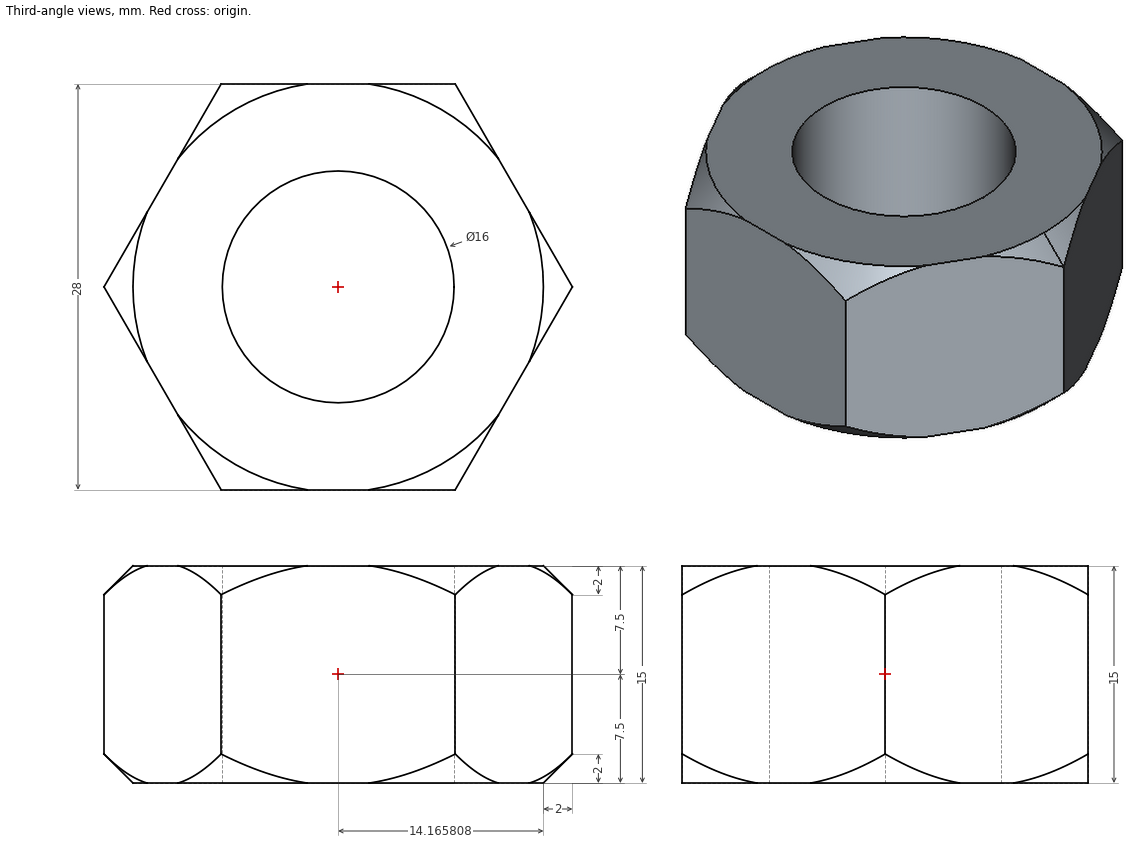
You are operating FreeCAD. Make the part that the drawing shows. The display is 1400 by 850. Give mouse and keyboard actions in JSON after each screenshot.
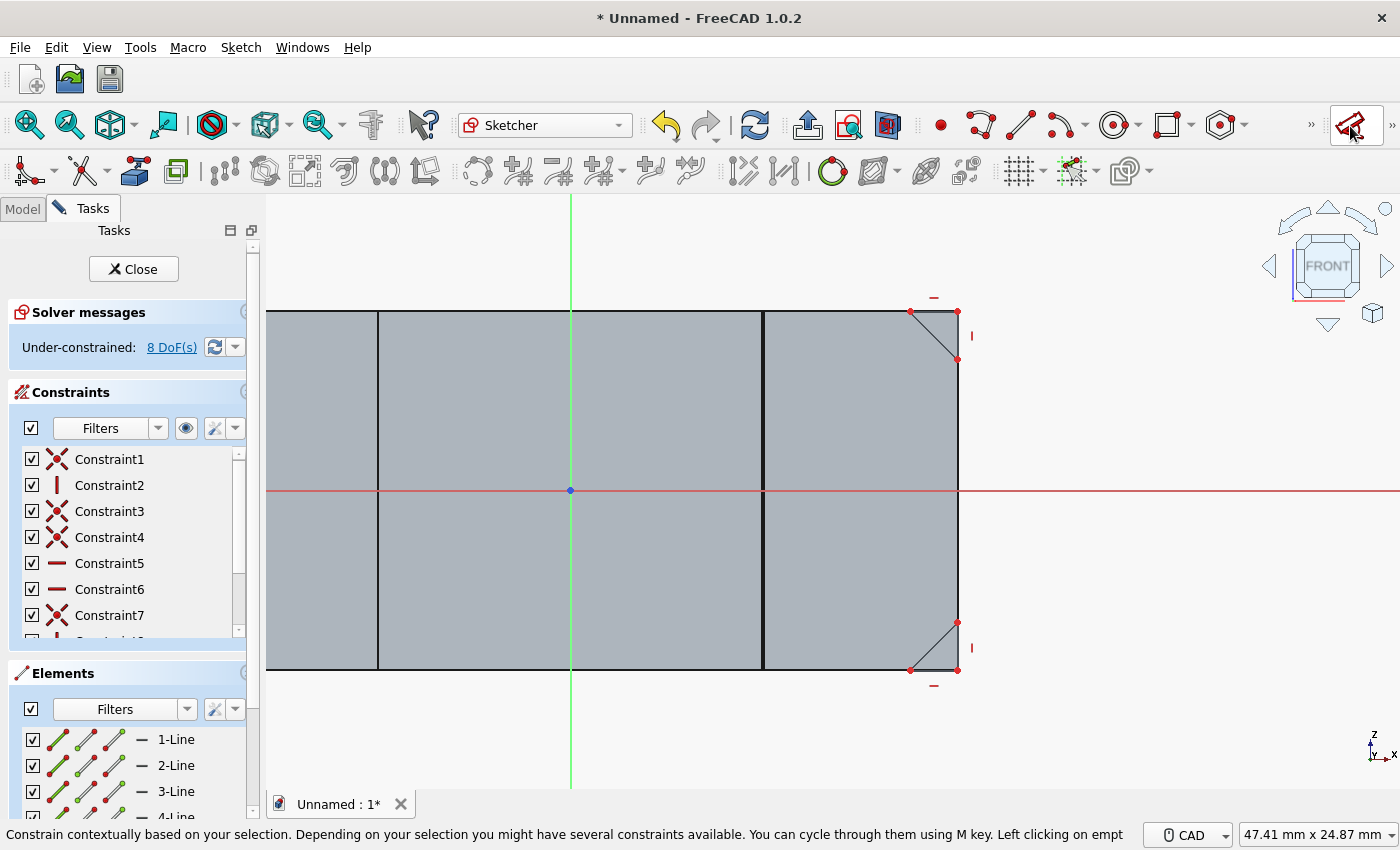
{"action": "scroll", "coordinate": [958, 637], "scroll_direction": "up", "scroll_amount": 2}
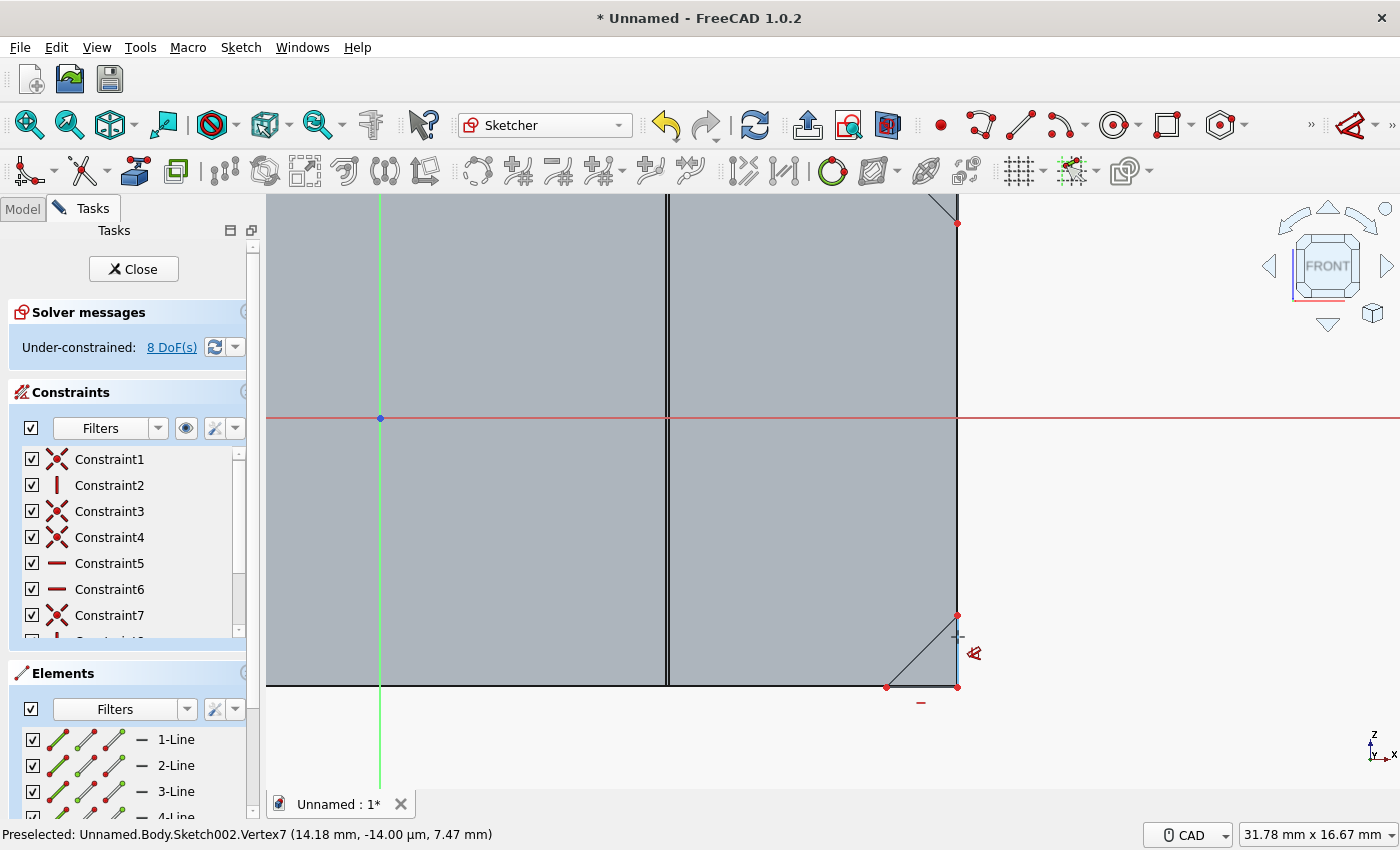
{"action": "left_click", "coordinate": [958, 637]}
{"action": "left_click", "coordinate": [992, 652]}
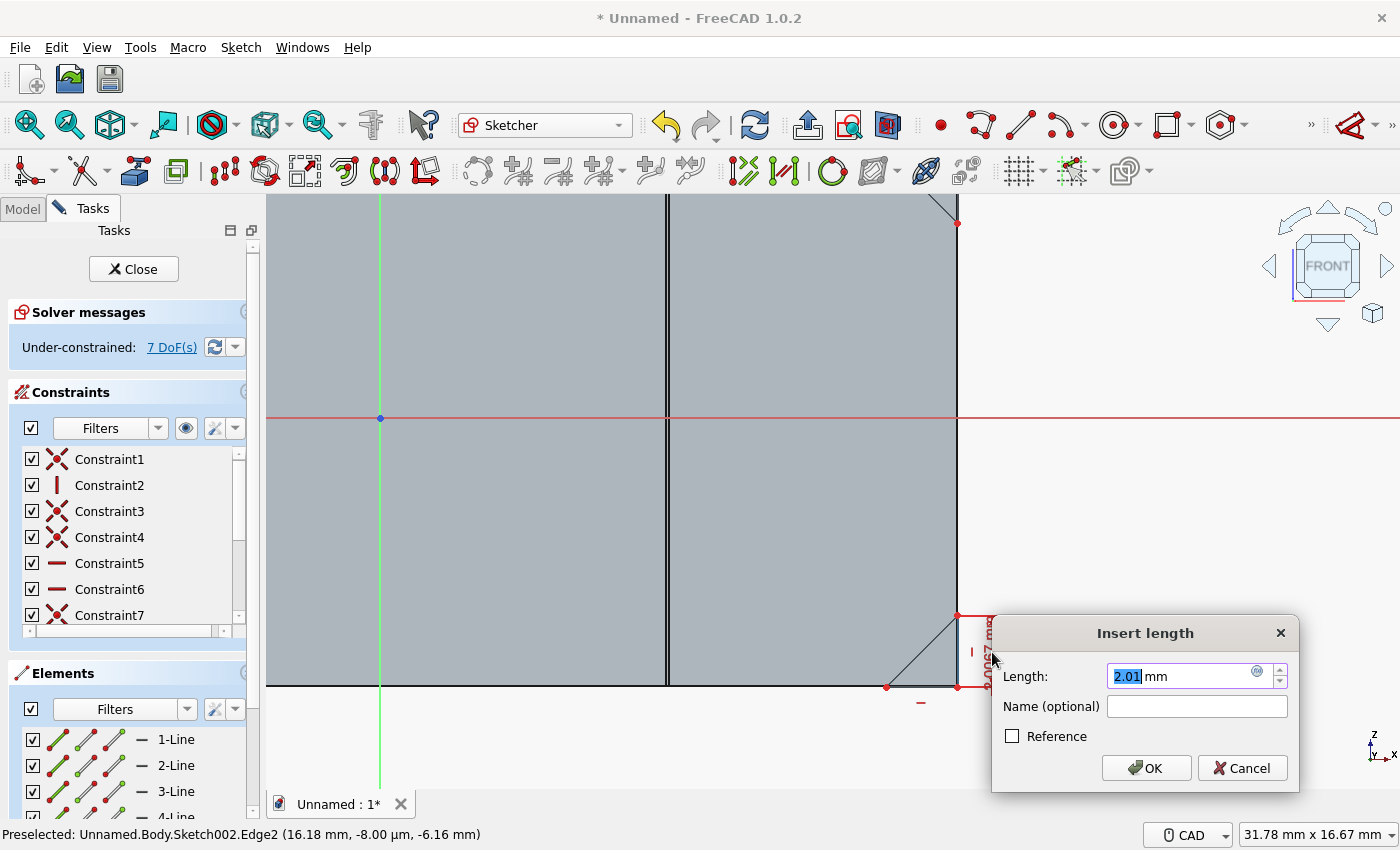
{"action": "type", "text": "2"}
{"action": "key", "text": "Return"}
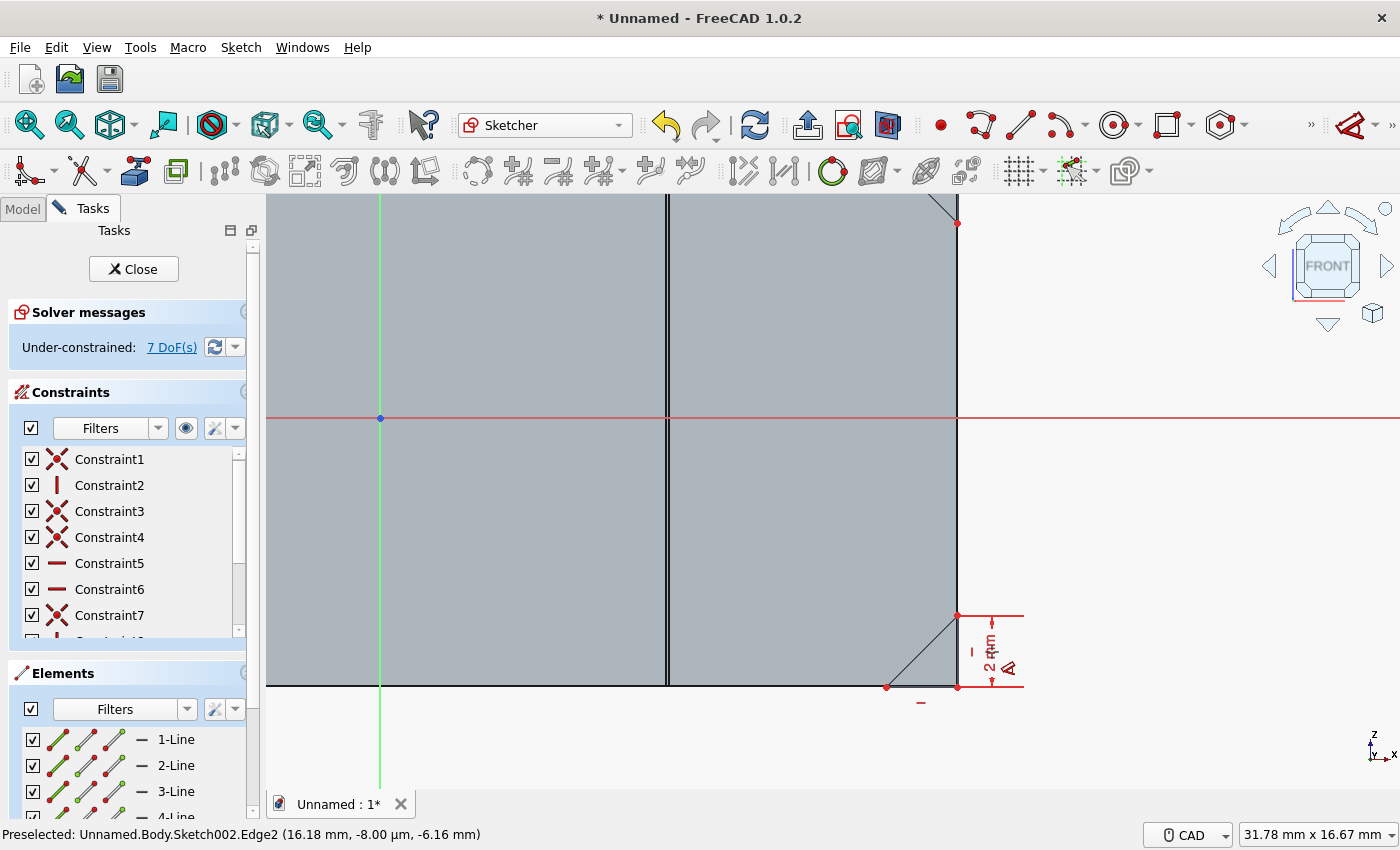
{"action": "left_click", "coordinate": [936, 687]}
{"action": "left_click", "coordinate": [922, 721]}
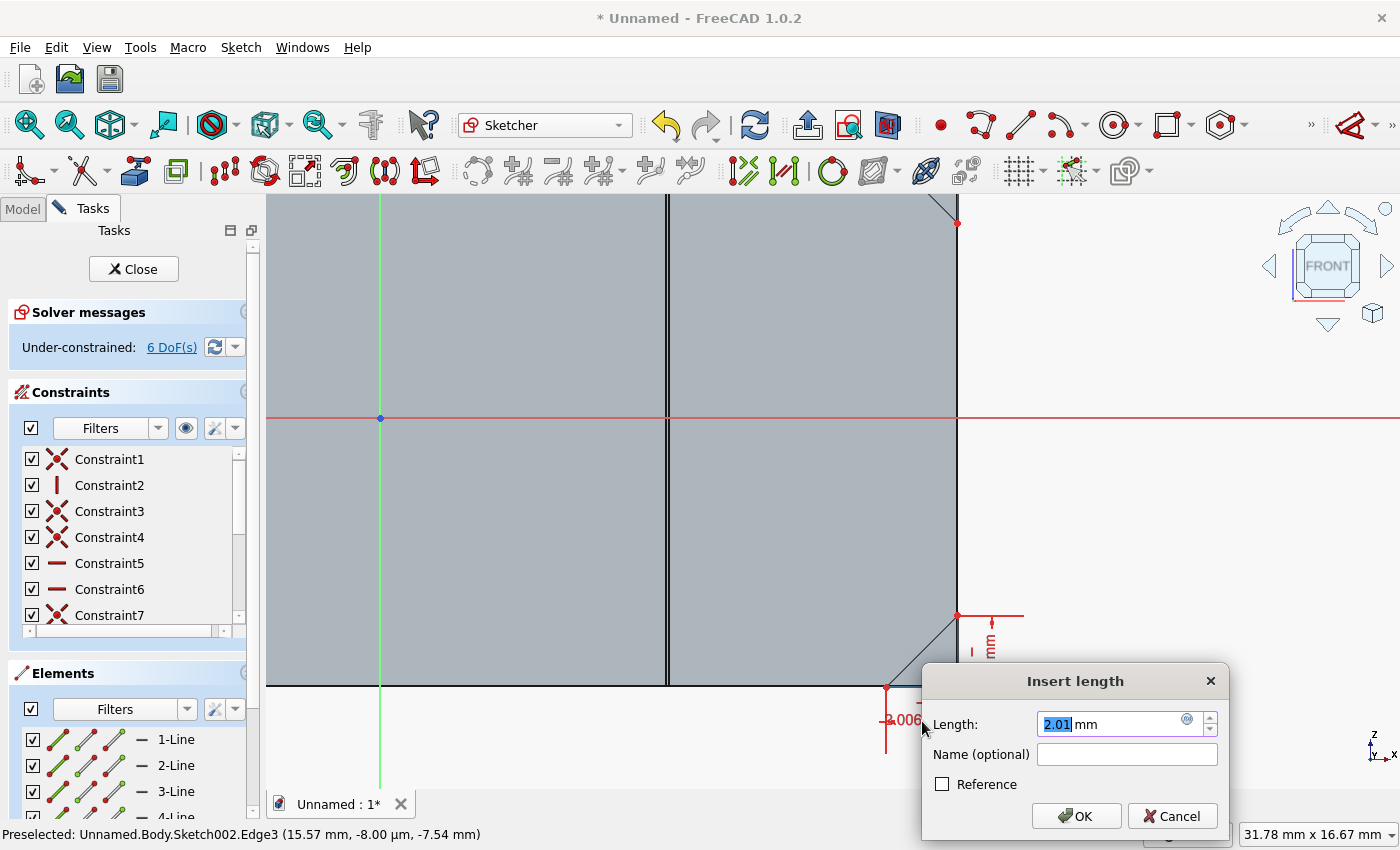
{"action": "type", "text": "2"}
{"action": "key", "text": "Return"}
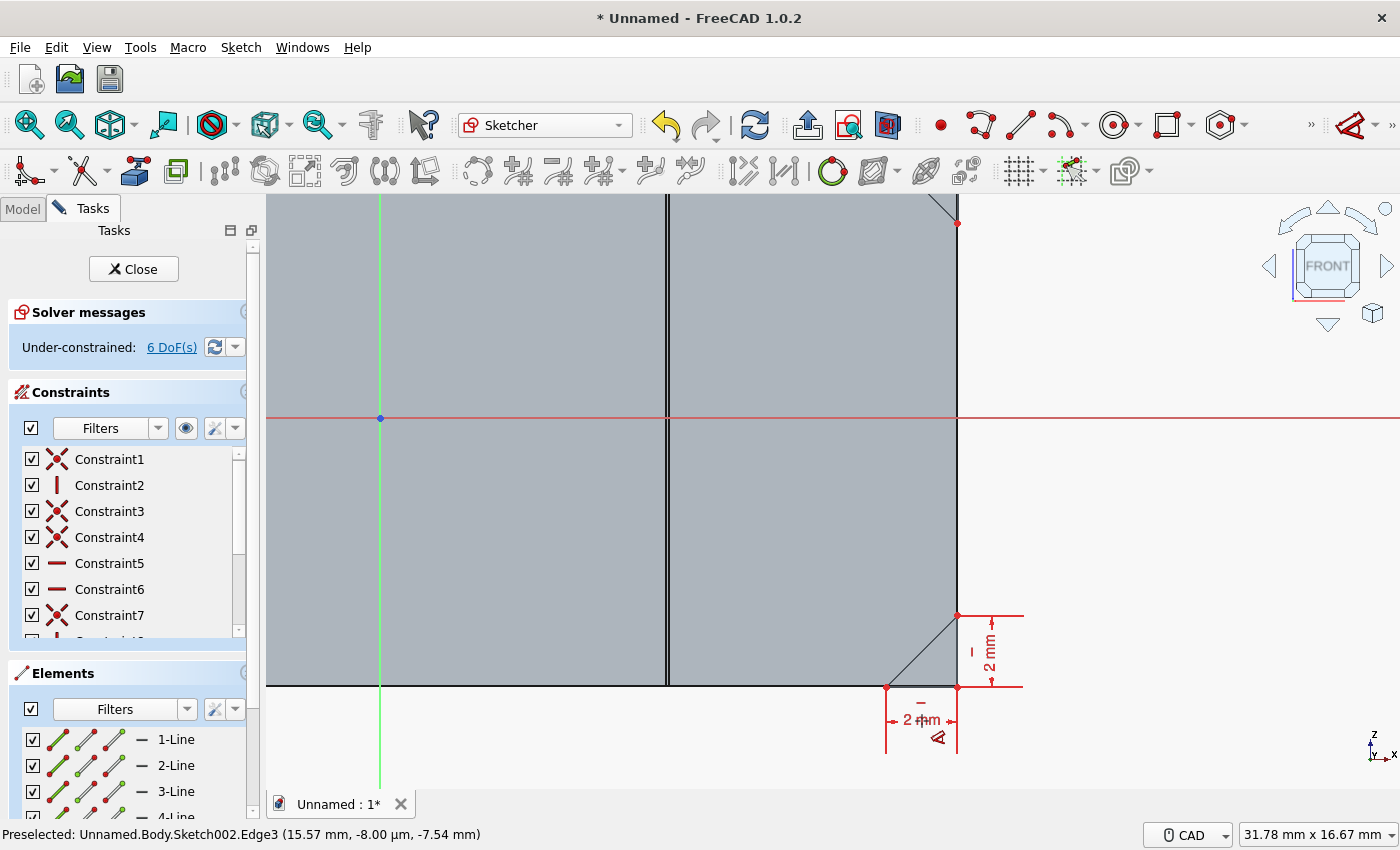
{"action": "scroll", "coordinate": [959, 640], "scroll_direction": "down", "scroll_amount": 2}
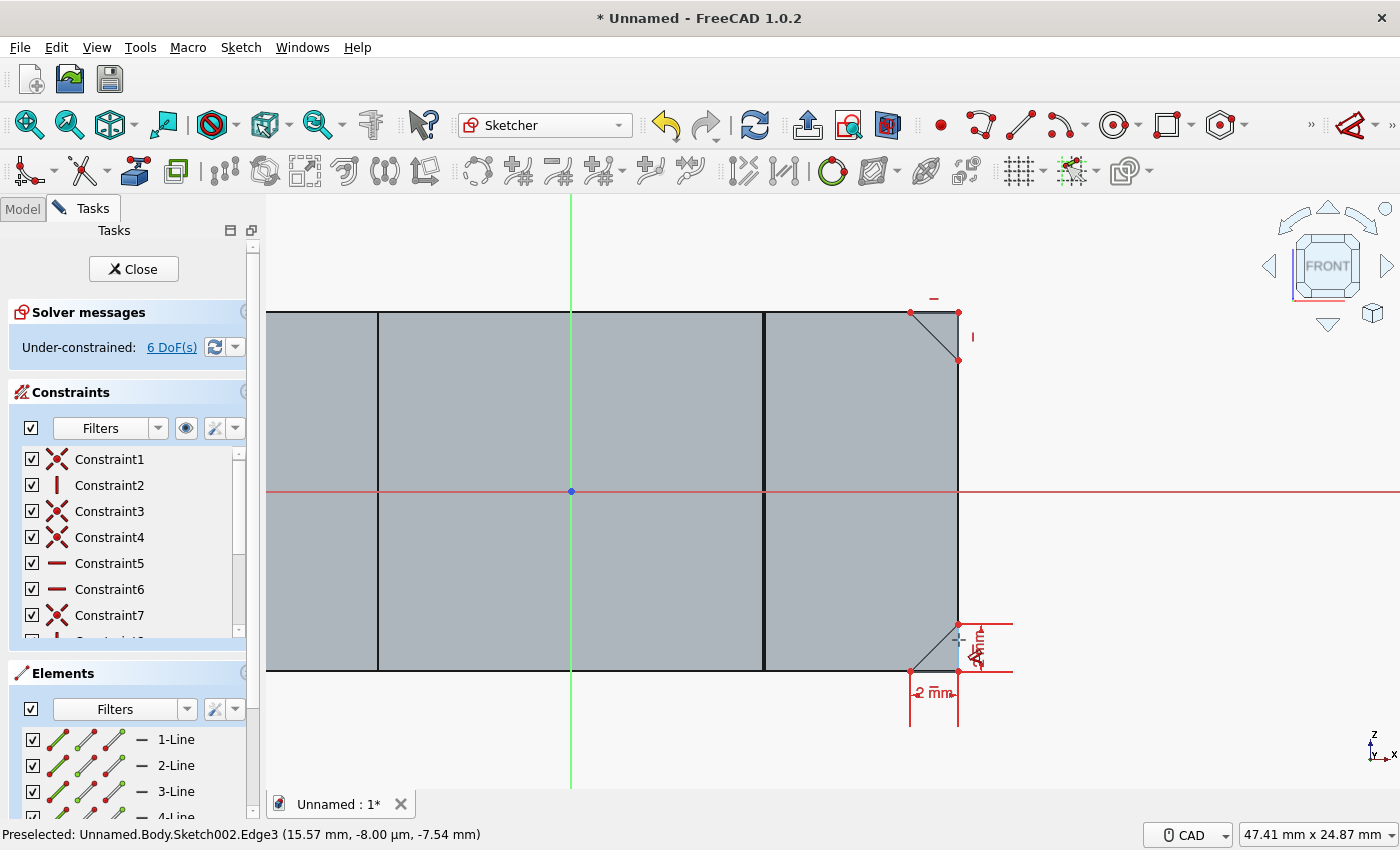
{"action": "scroll", "coordinate": [925, 313], "scroll_direction": "up", "scroll_amount": 2}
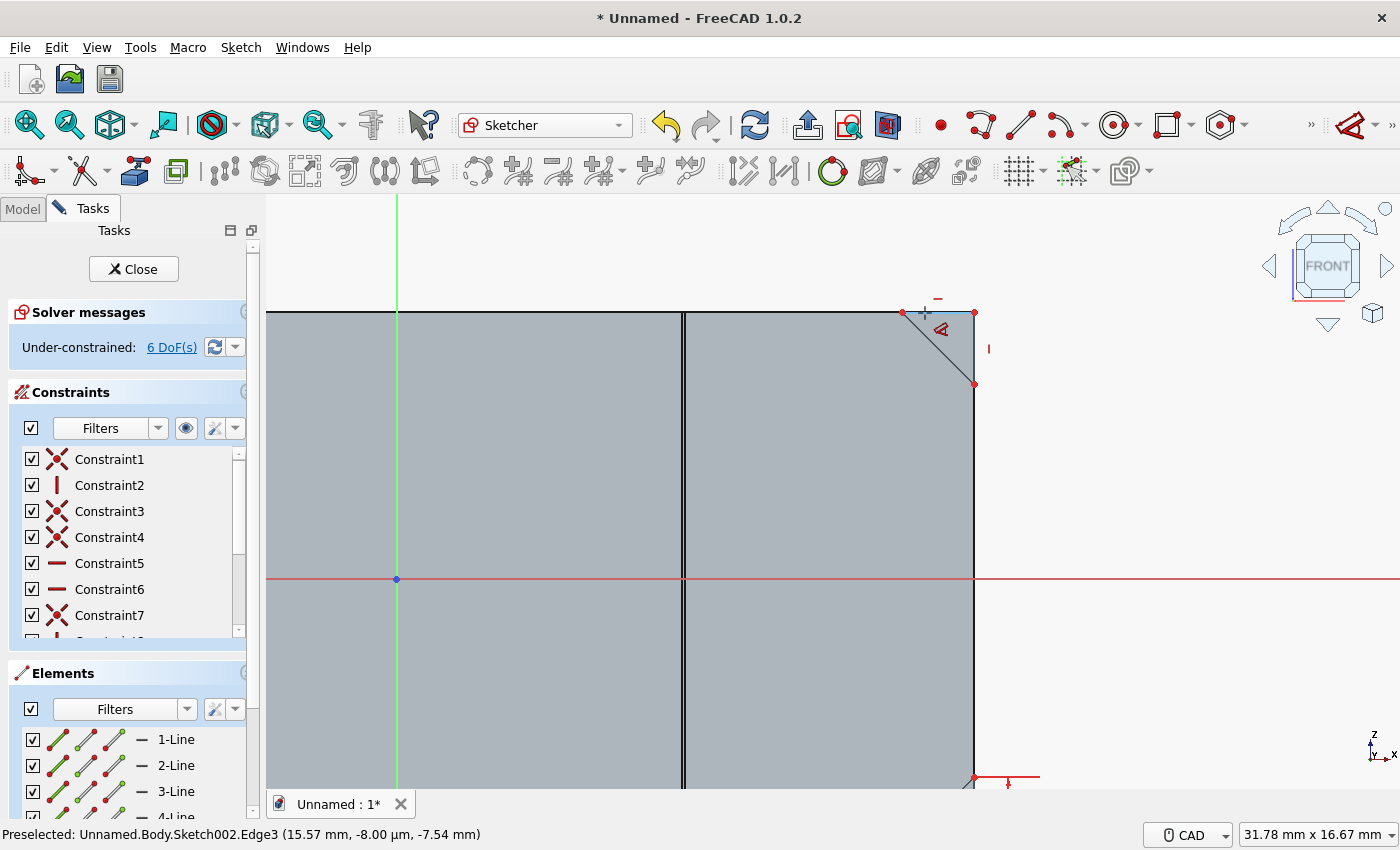
{"action": "left_click", "coordinate": [924, 313]}
{"action": "left_click", "coordinate": [939, 279]}